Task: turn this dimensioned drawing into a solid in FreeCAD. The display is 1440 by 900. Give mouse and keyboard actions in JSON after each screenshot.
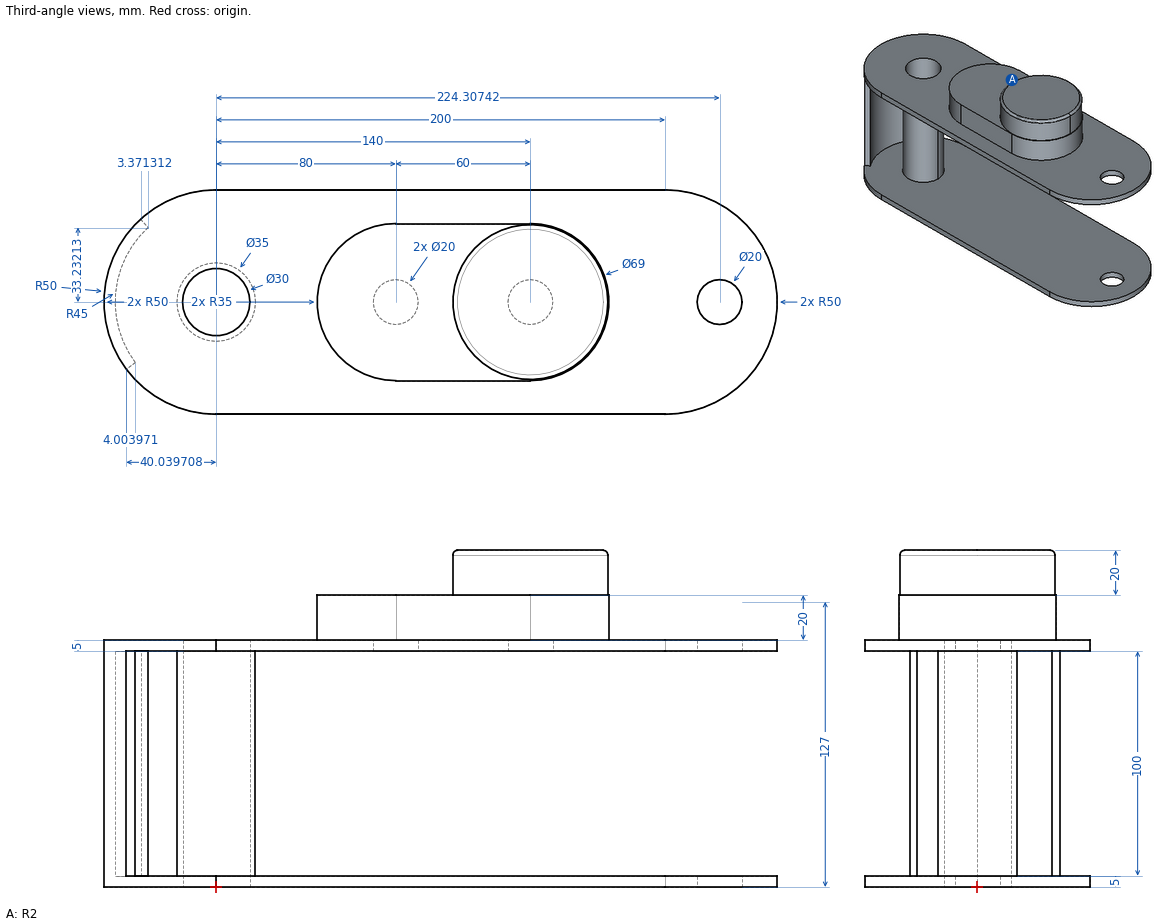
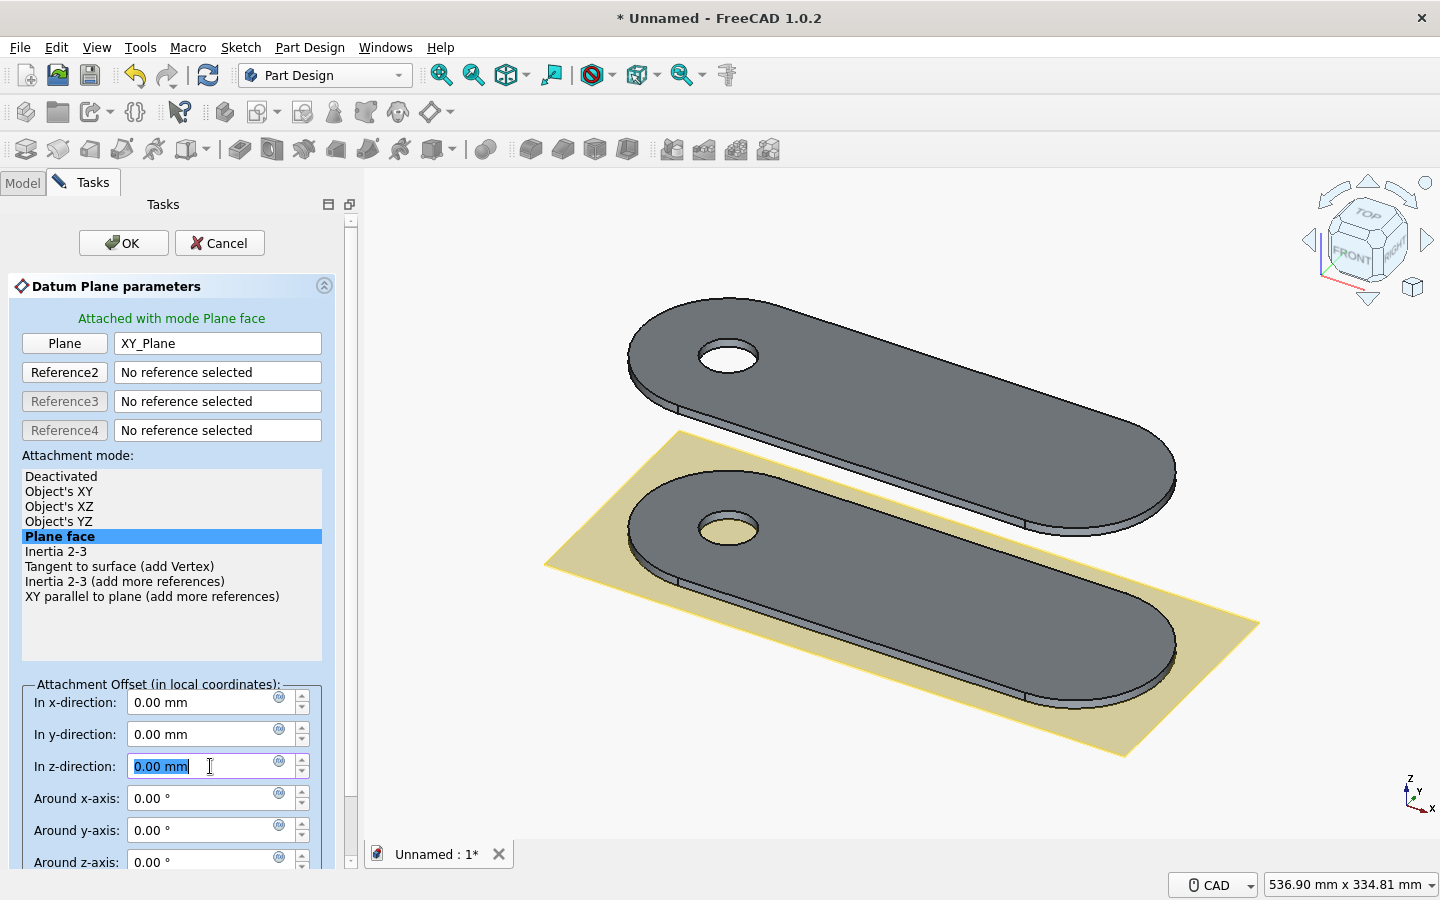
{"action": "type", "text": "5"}
{"action": "key", "text": "Tab"}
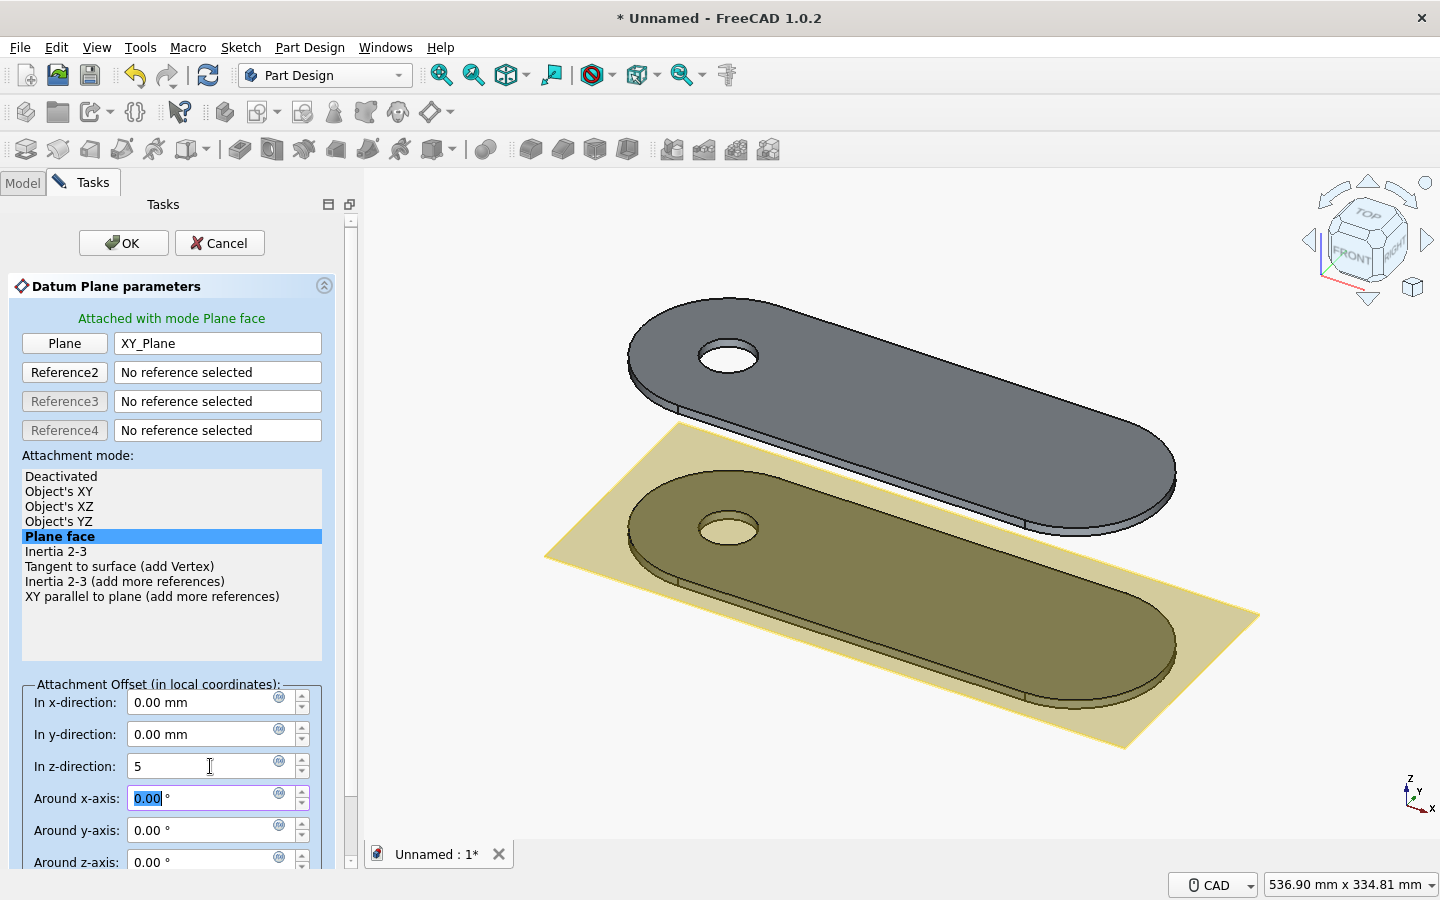
{"action": "left_click", "coordinate": [124, 243]}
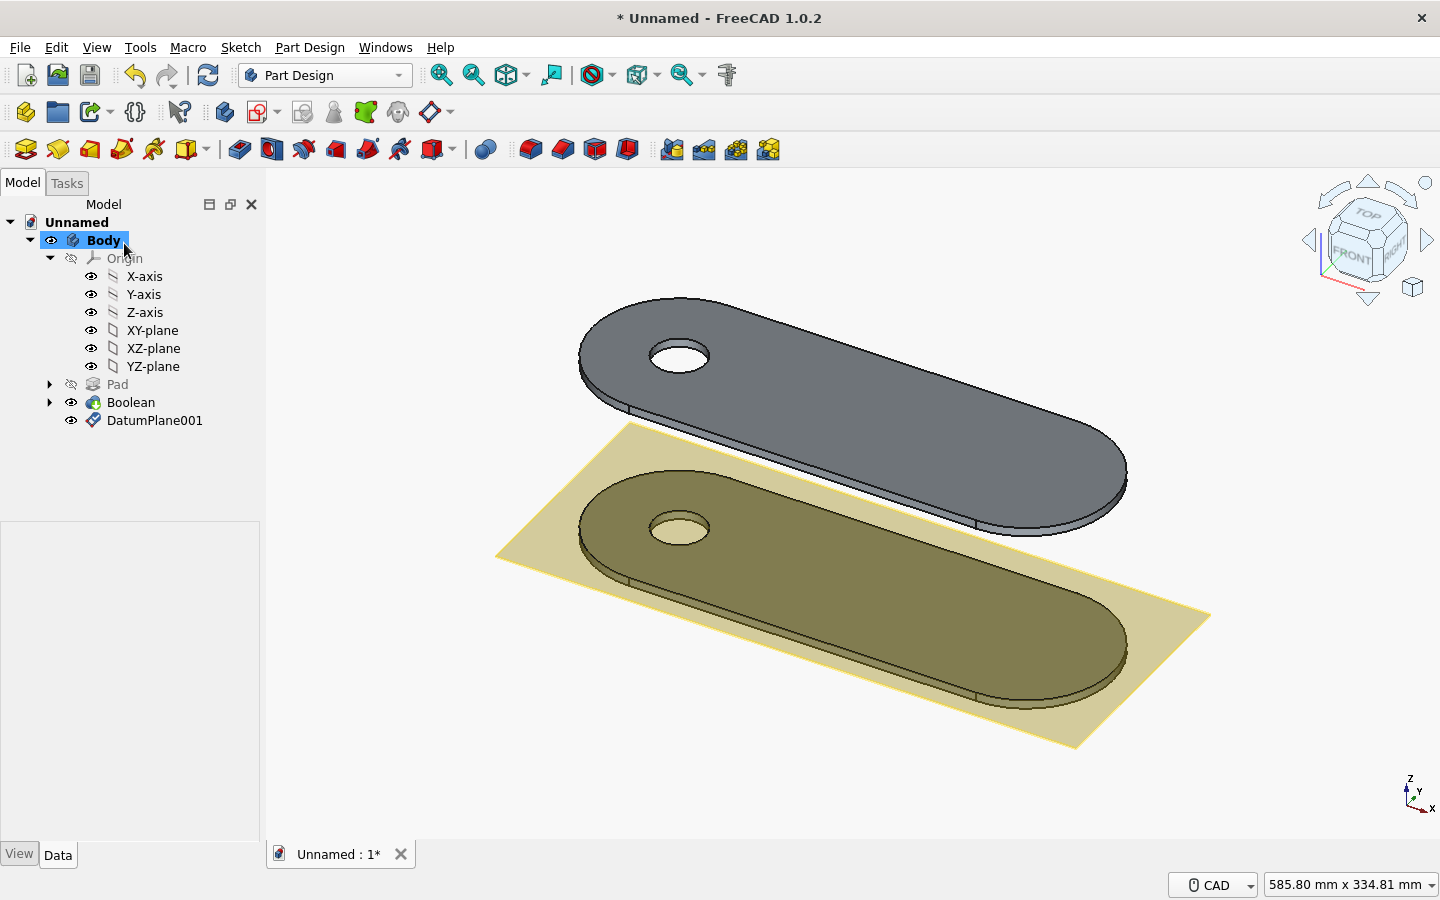
{"action": "left_click", "coordinate": [116, 420]}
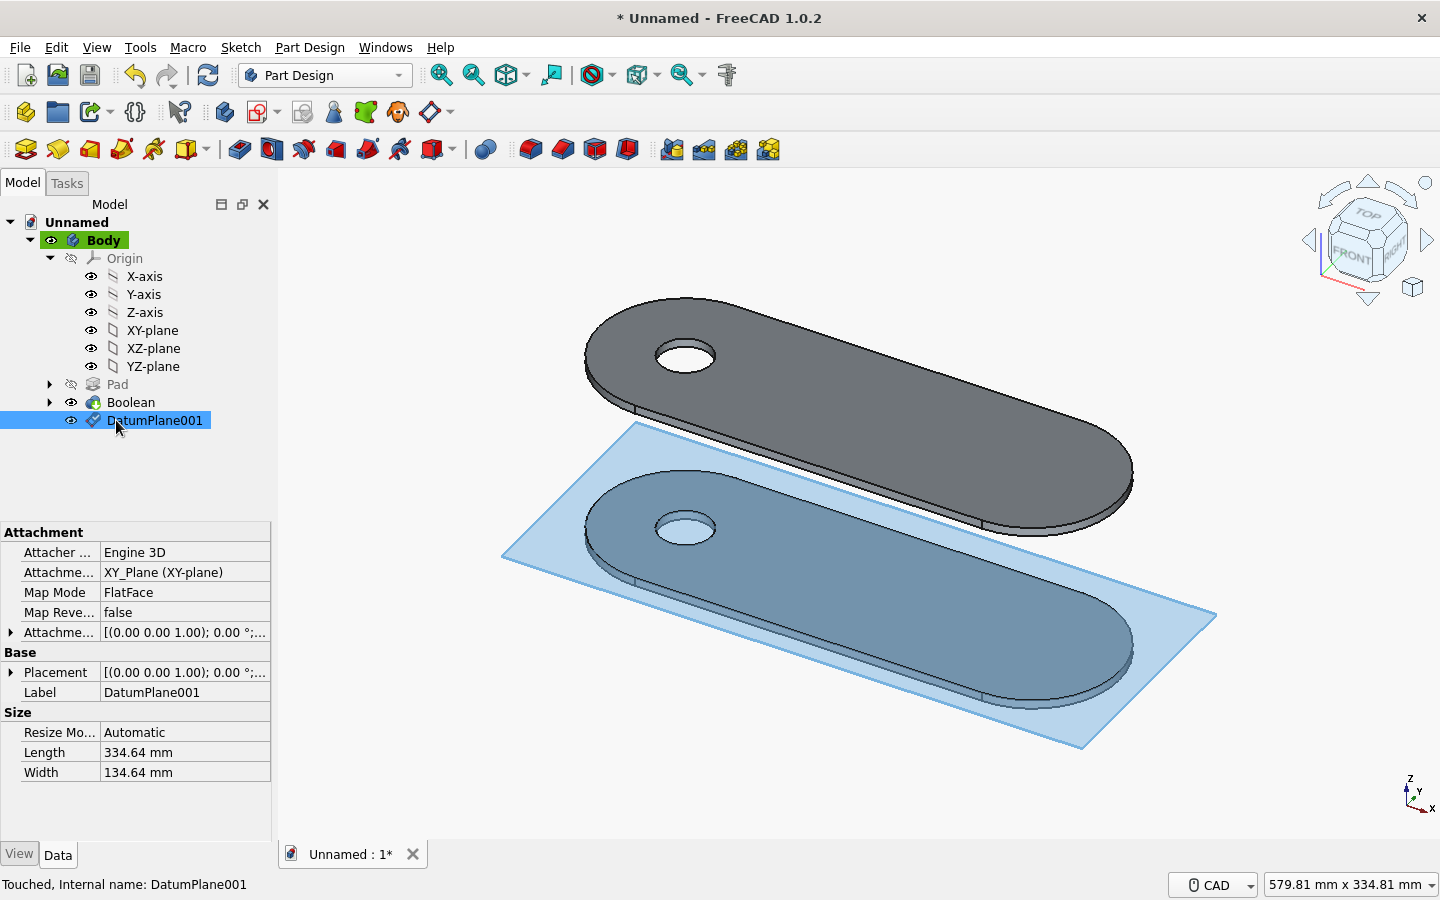
{"action": "left_click", "coordinate": [258, 112]}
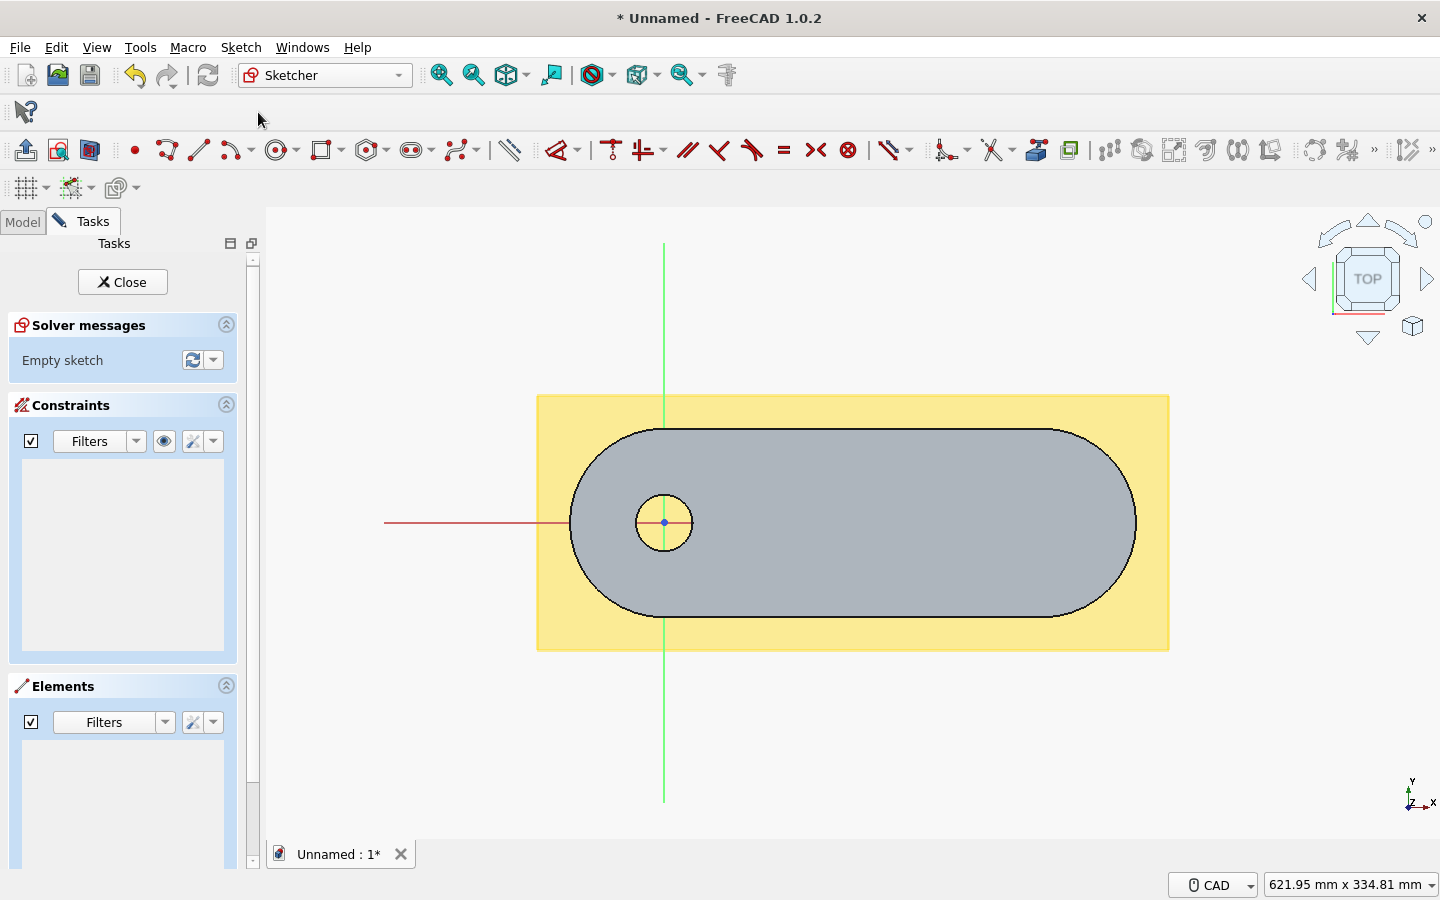
{"action": "left_click", "coordinate": [90, 150]}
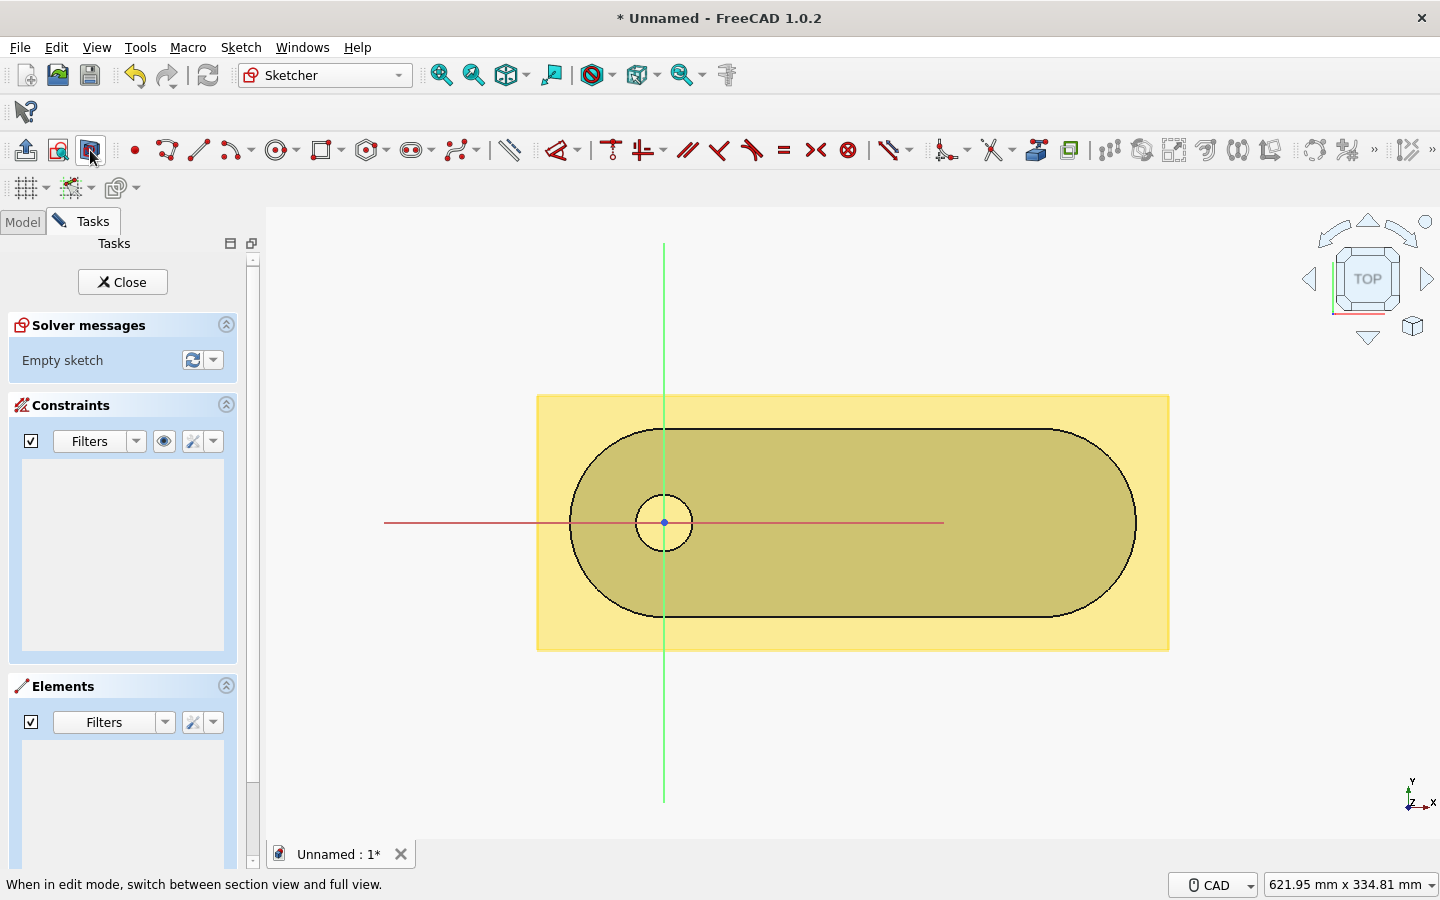
{"action": "scroll", "coordinate": [640, 523], "scroll_direction": "up", "scroll_amount": 9}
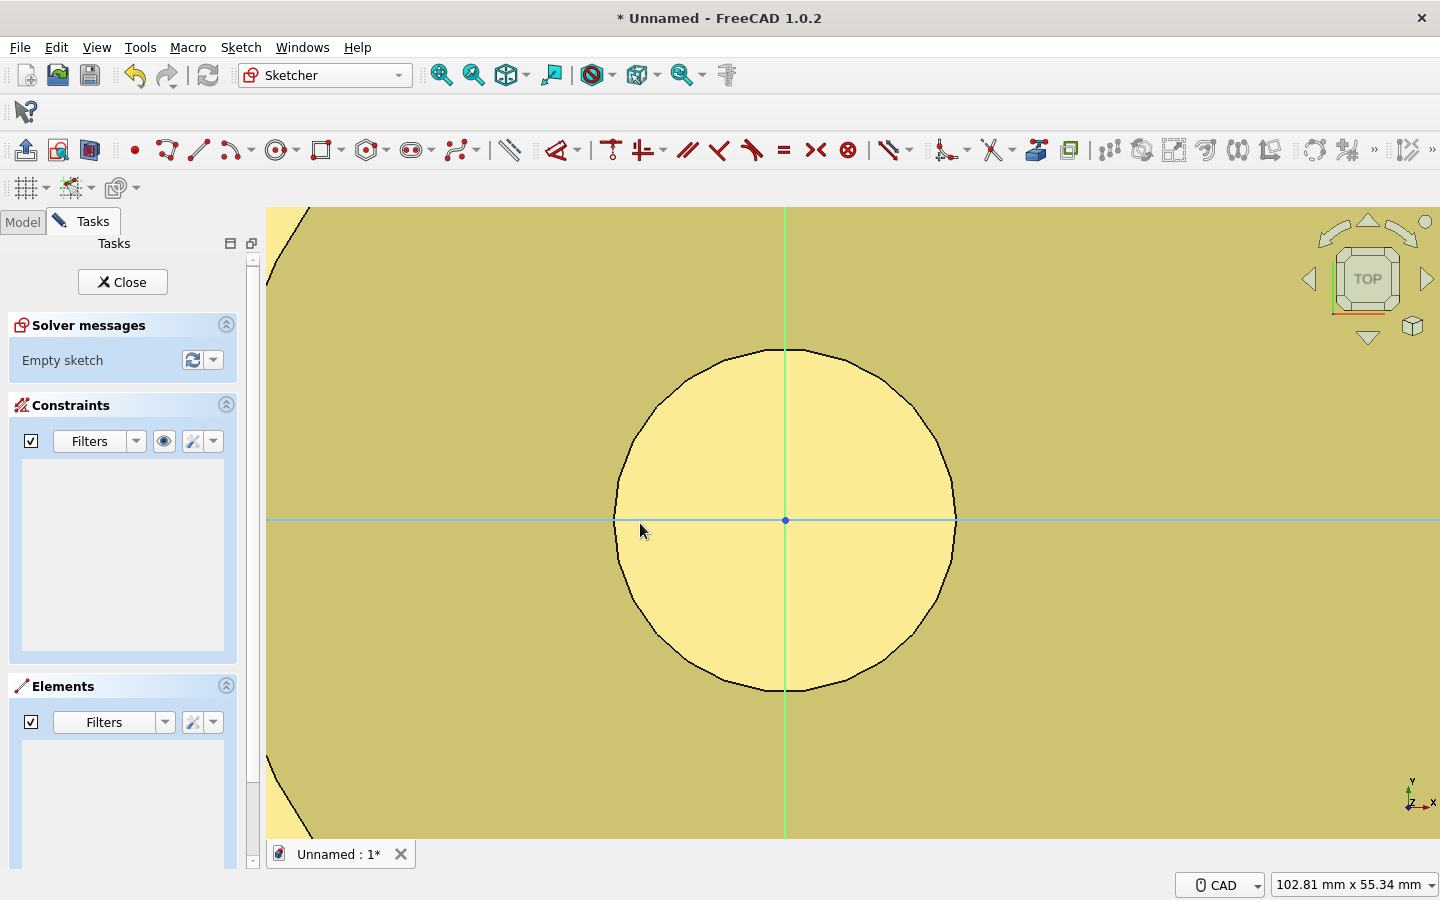
{"action": "left_click", "coordinate": [276, 150]}